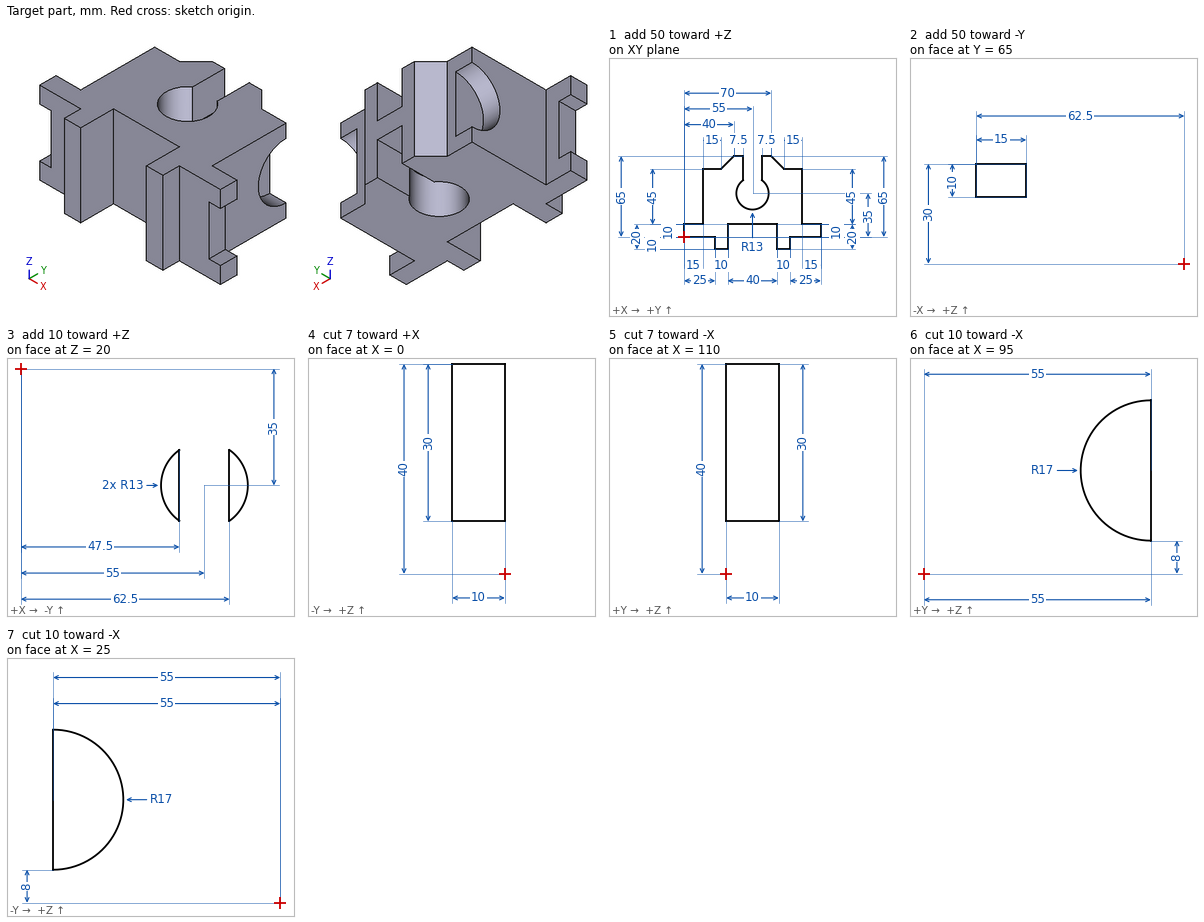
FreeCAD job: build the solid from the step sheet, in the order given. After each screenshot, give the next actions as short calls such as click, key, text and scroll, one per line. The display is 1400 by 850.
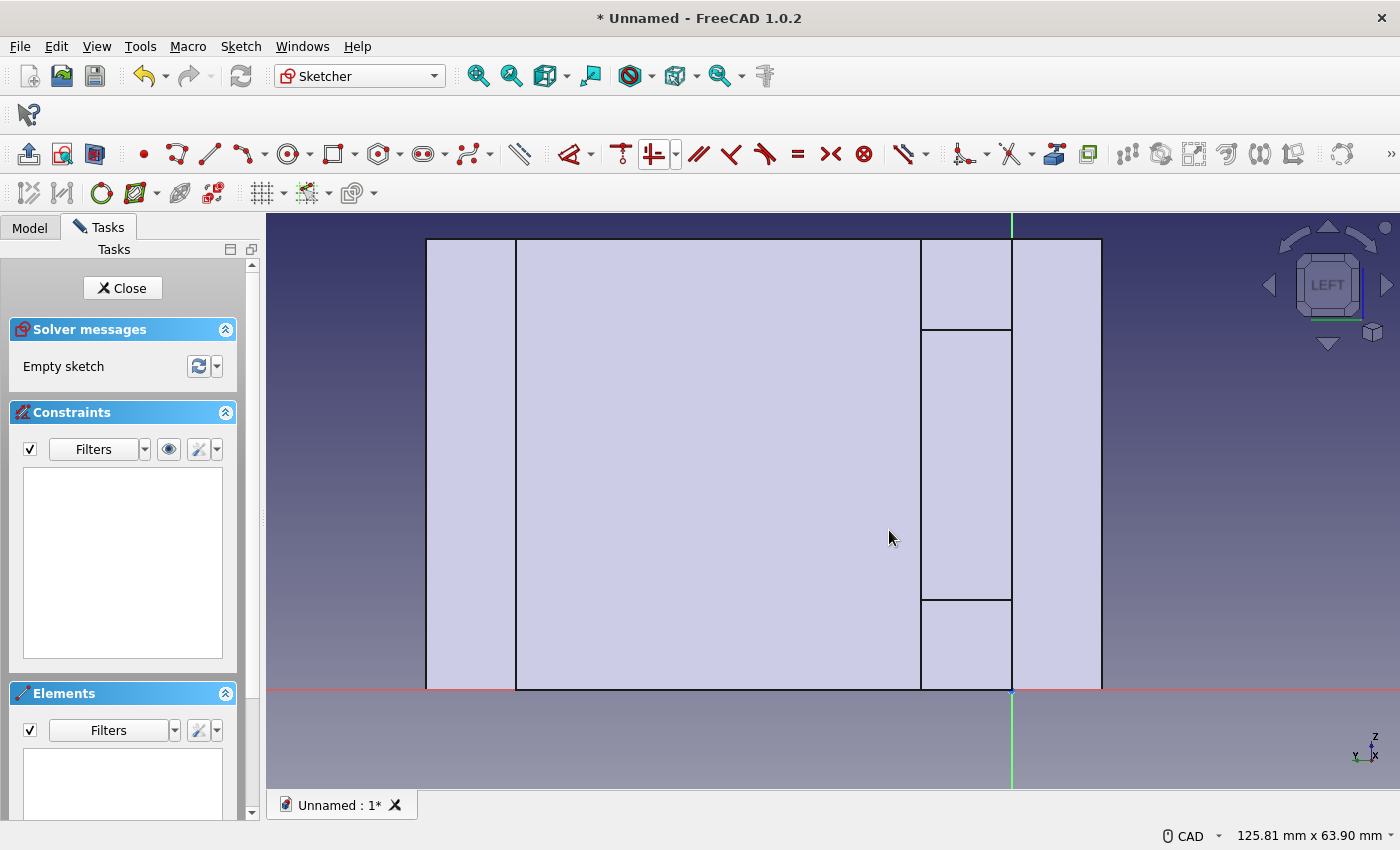
click(210, 154)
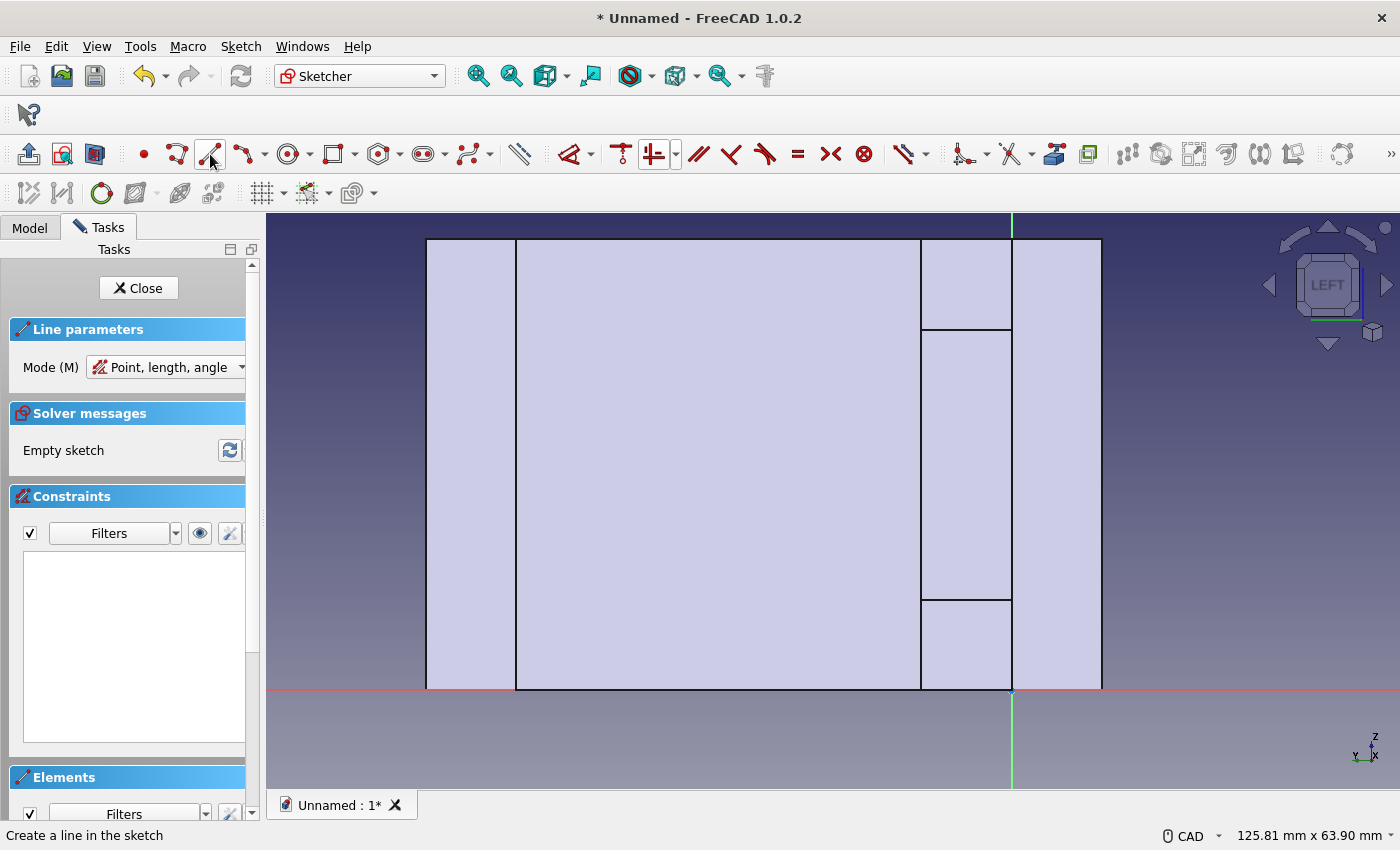
click(516, 312)
click(516, 618)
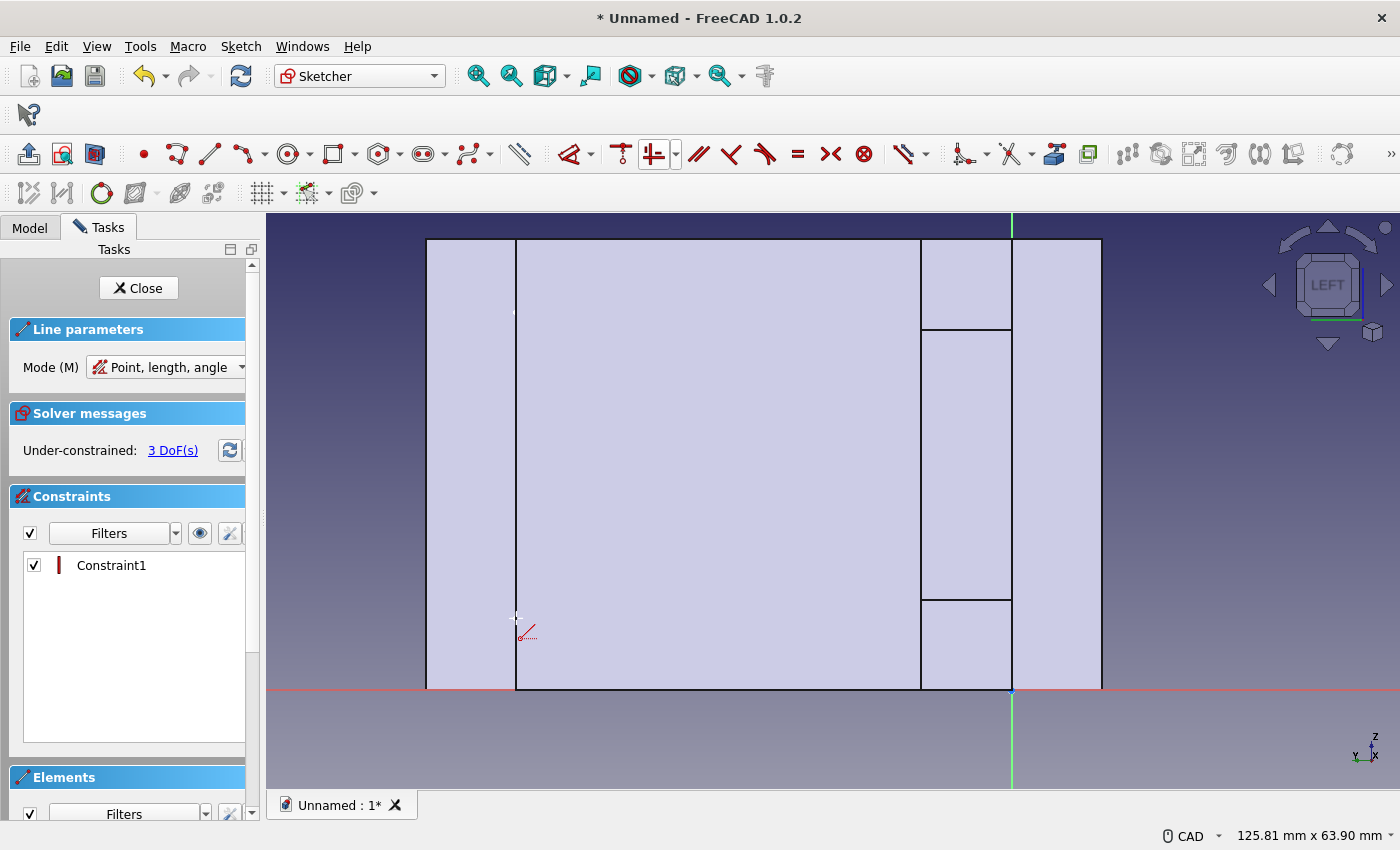
click(242, 154)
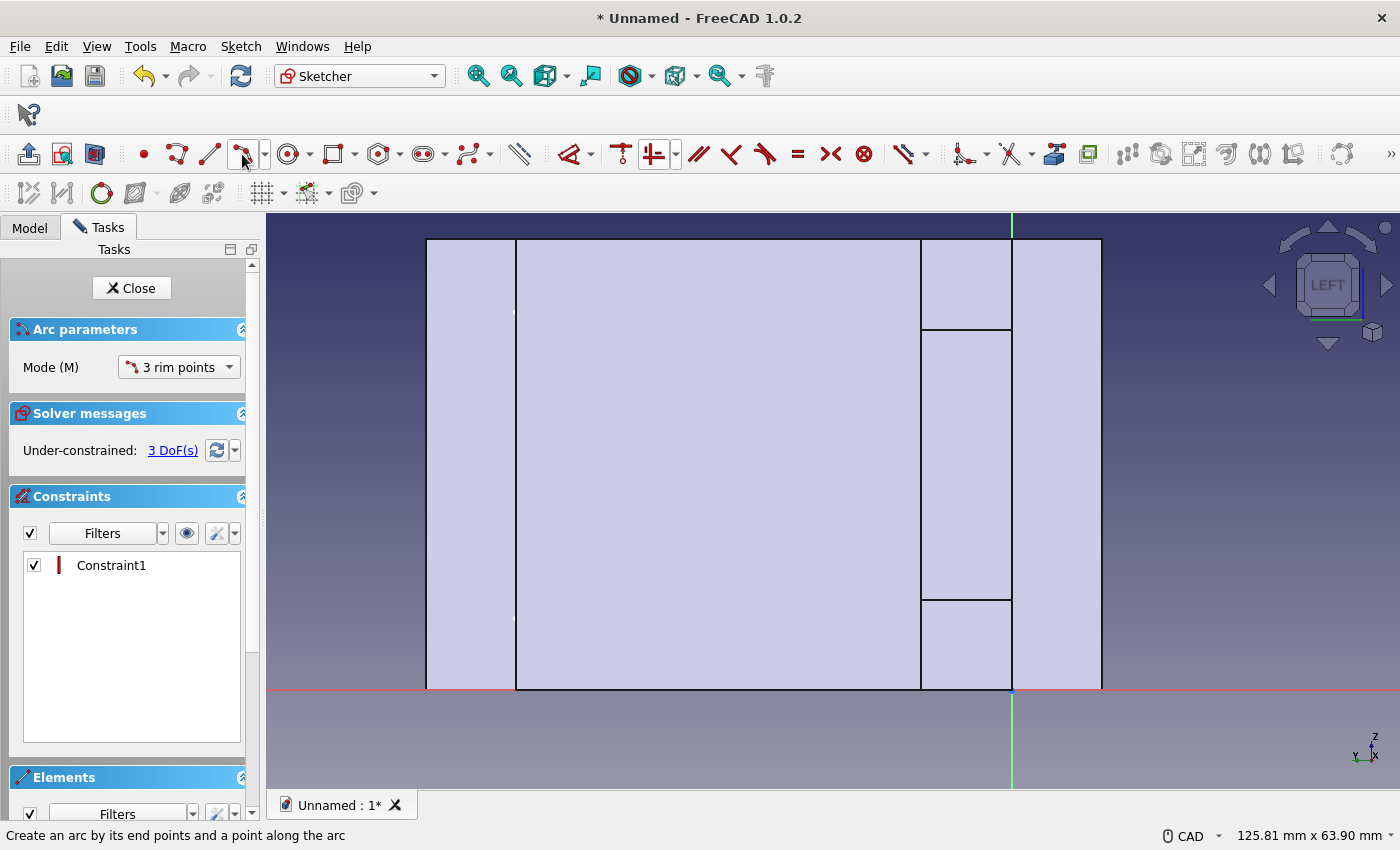
click(516, 619)
click(516, 313)
click(669, 465)
key(Escape)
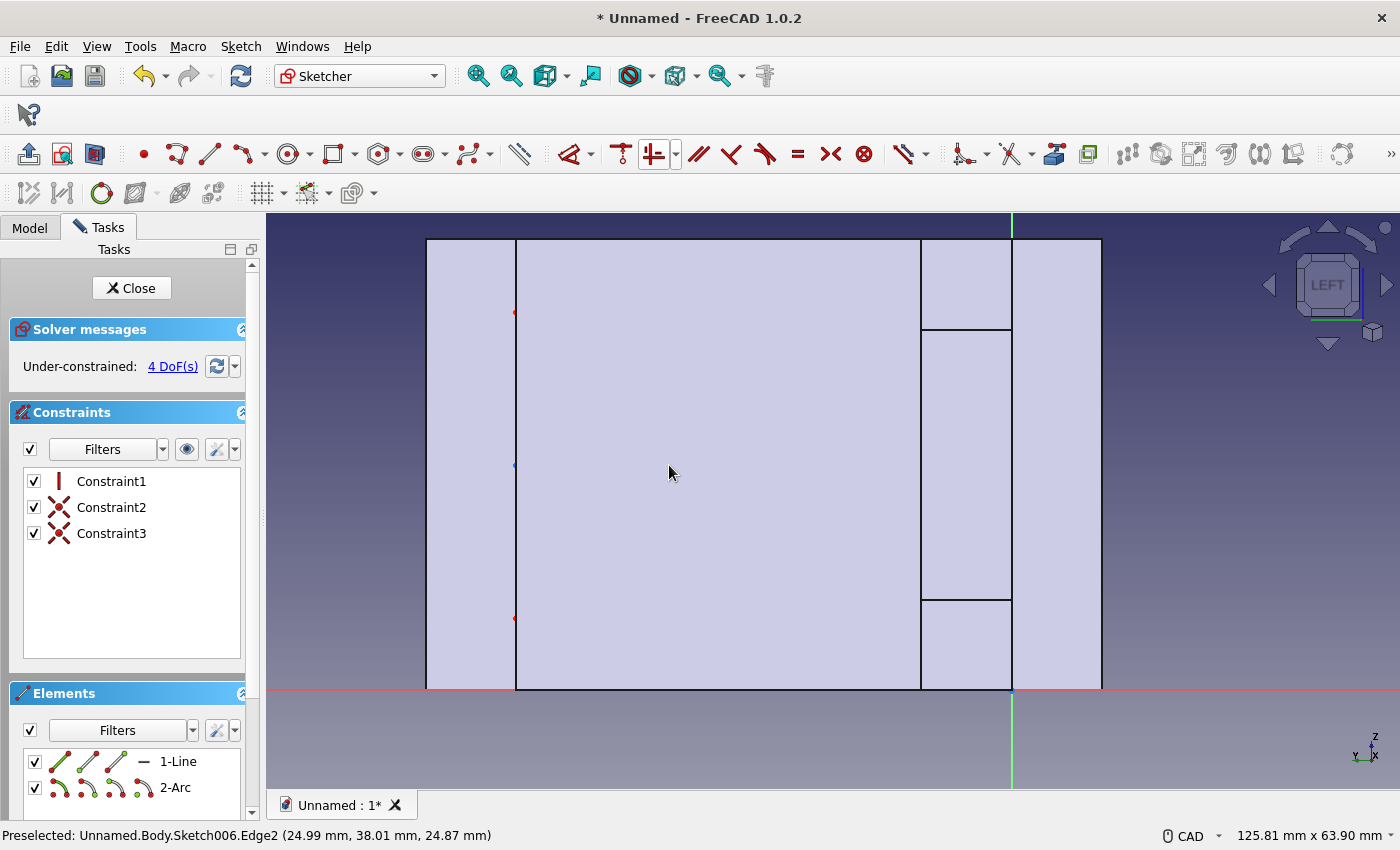
click(568, 154)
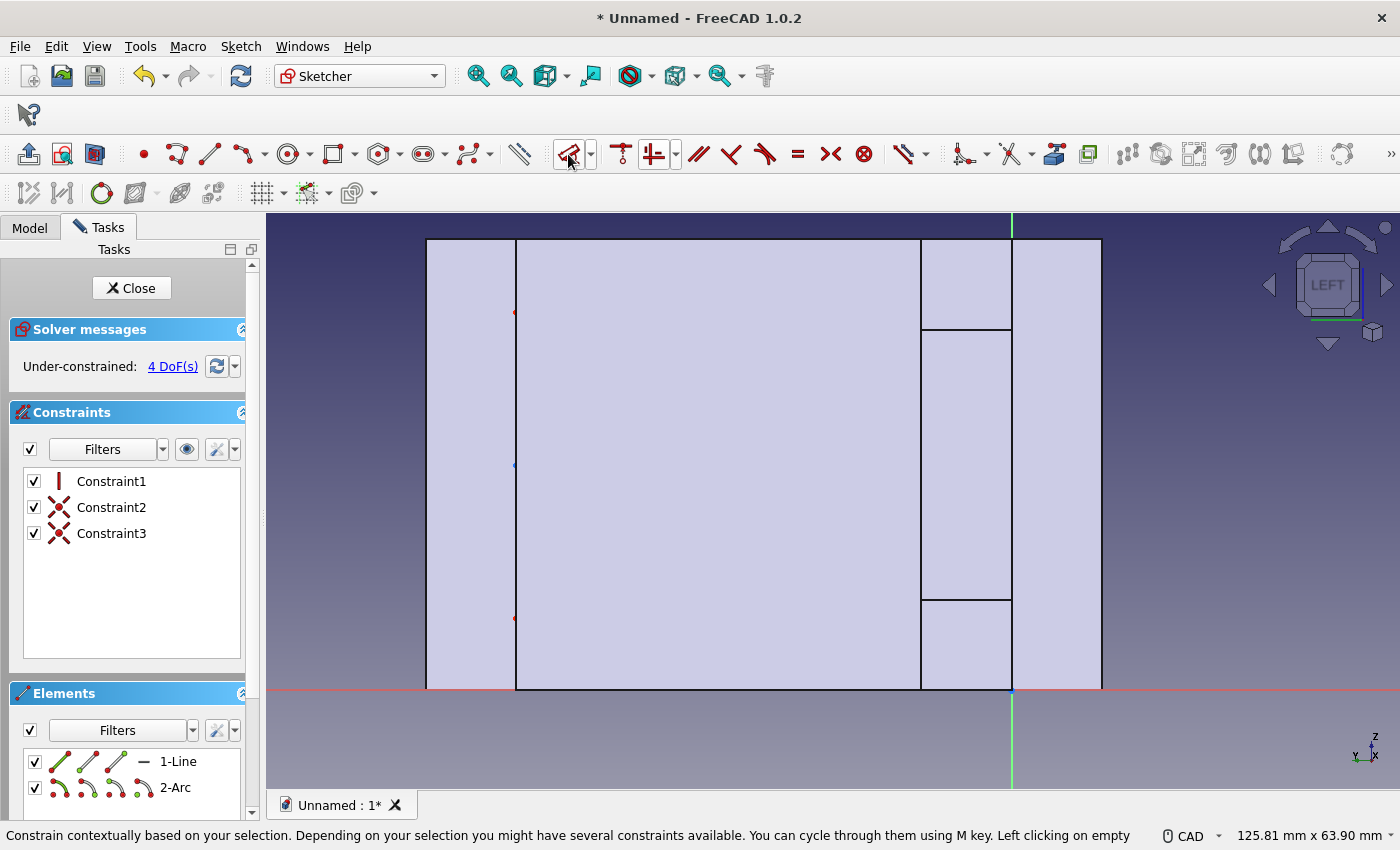
click(640, 556)
click(666, 575)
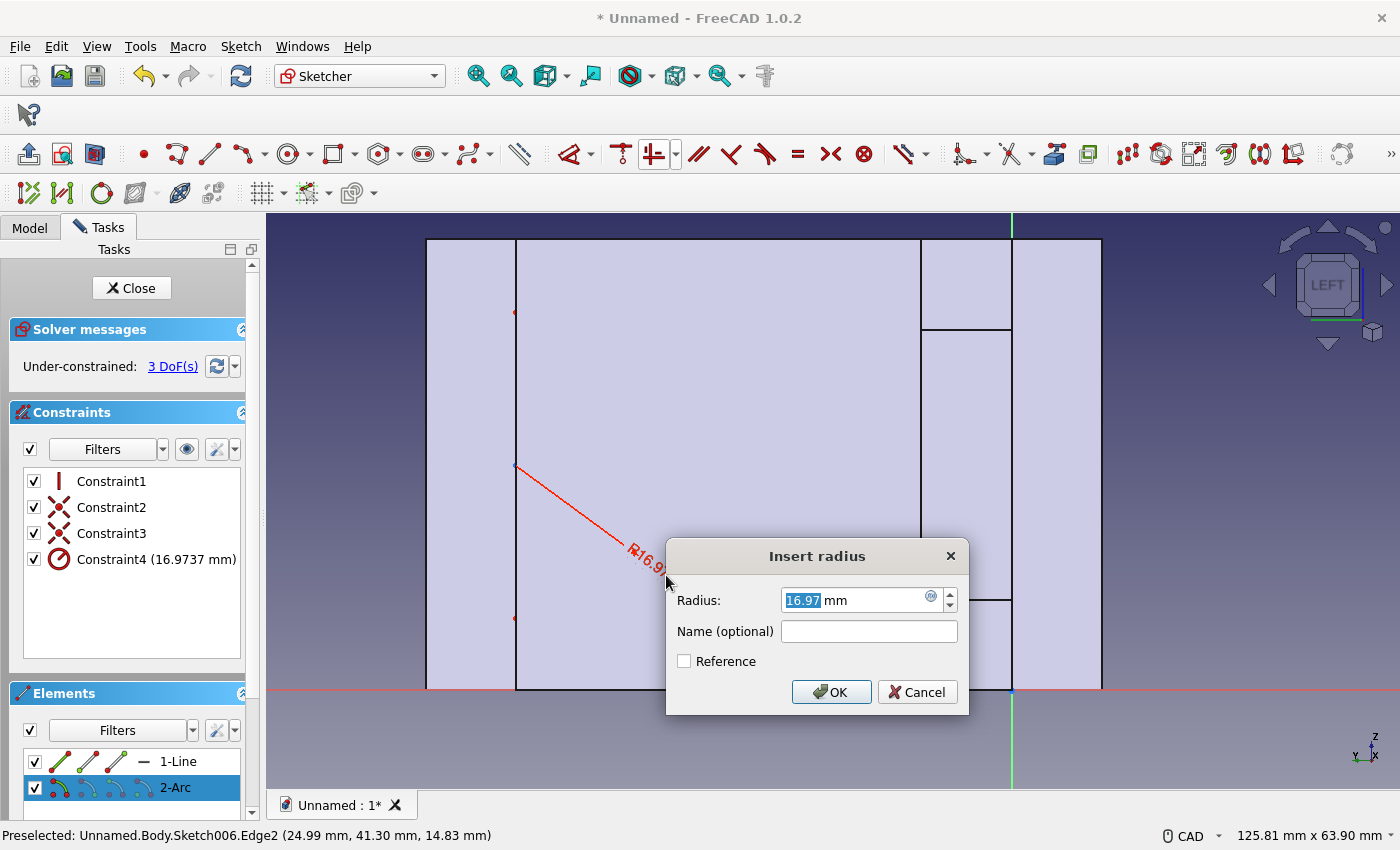
text(17)
key(Return)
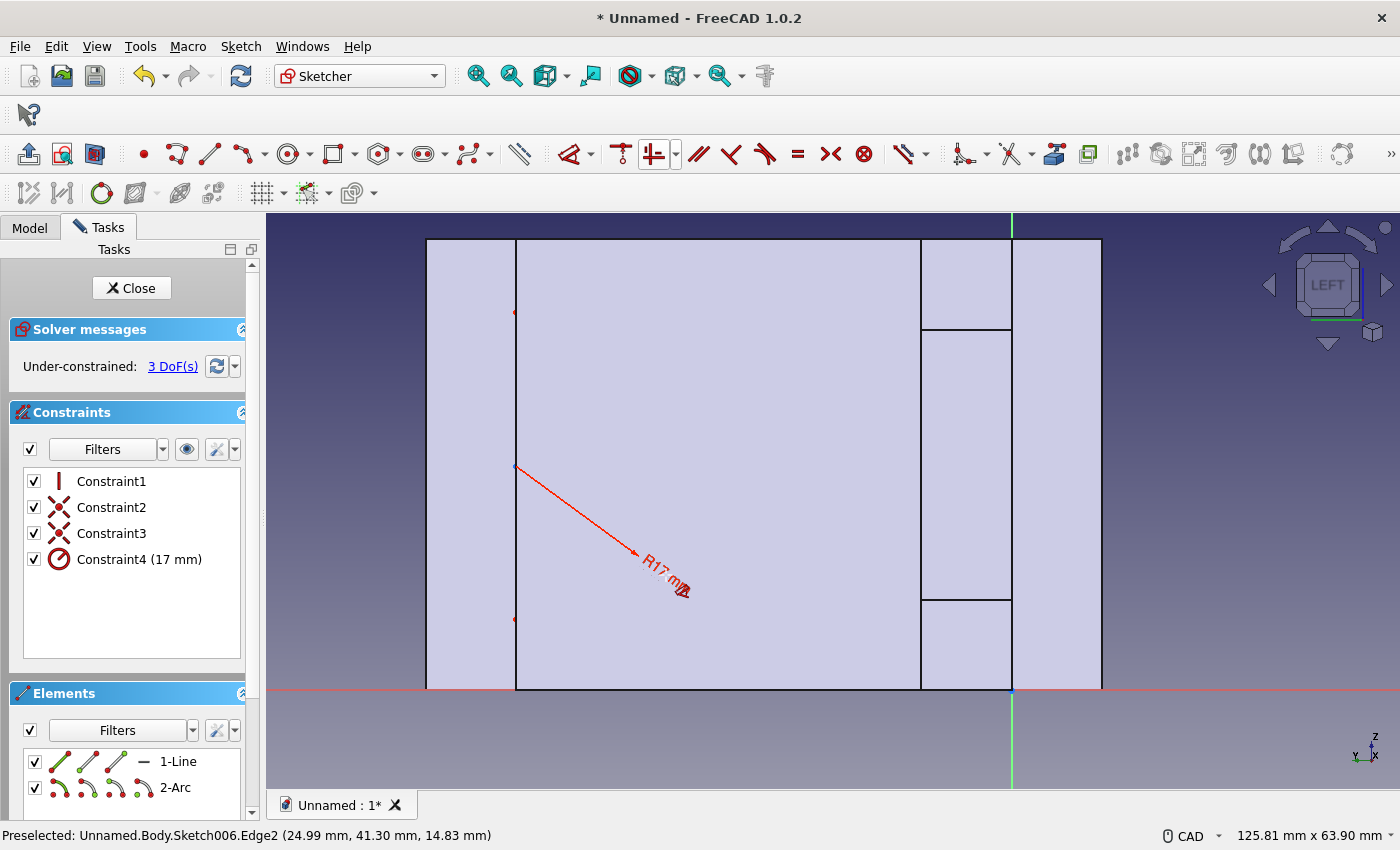
click(516, 619)
click(1046, 655)